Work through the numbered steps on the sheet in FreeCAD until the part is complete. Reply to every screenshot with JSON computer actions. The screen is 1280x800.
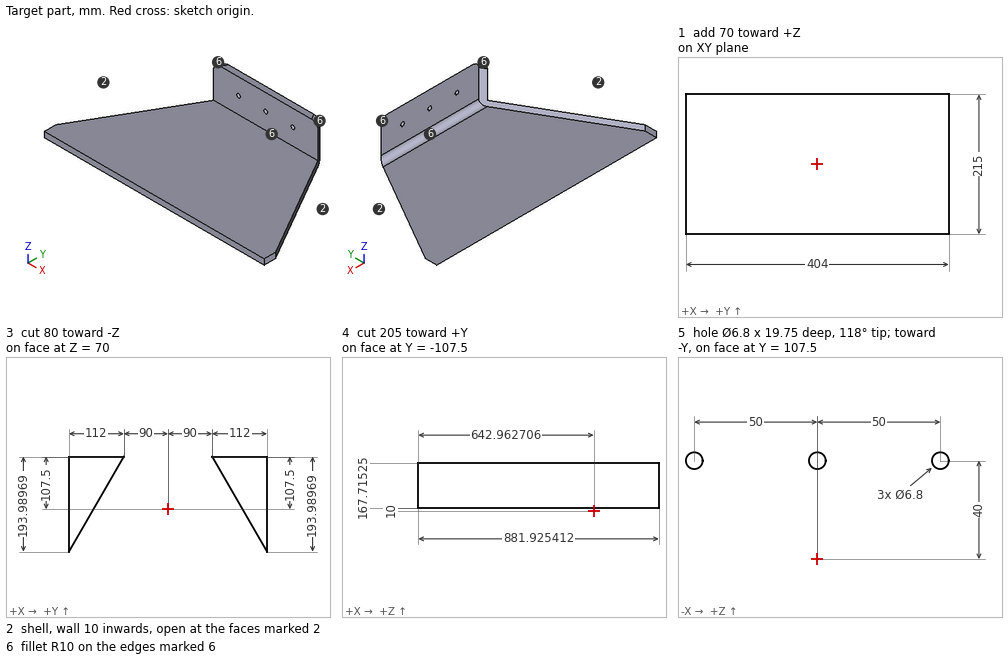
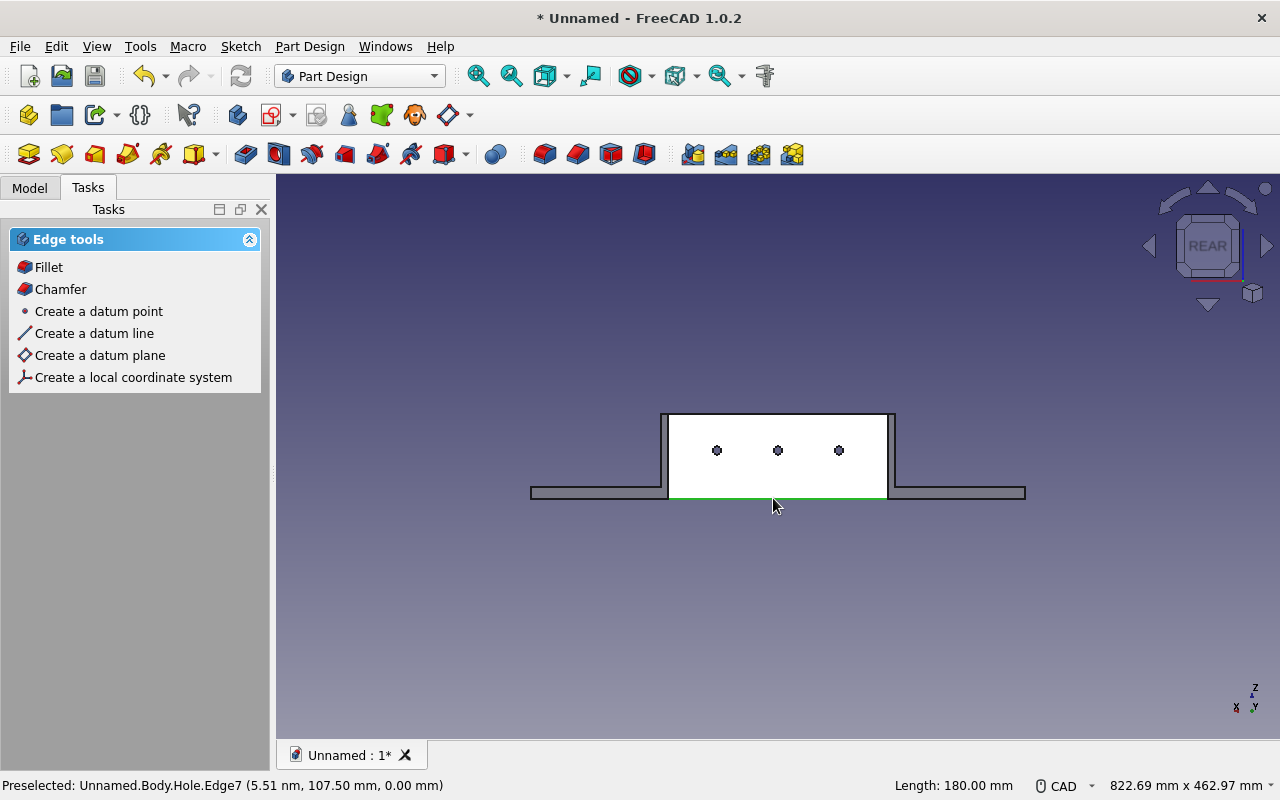
{"action": "scroll", "coordinate": [665, 413], "scroll_direction": "up", "scroll_amount": 6}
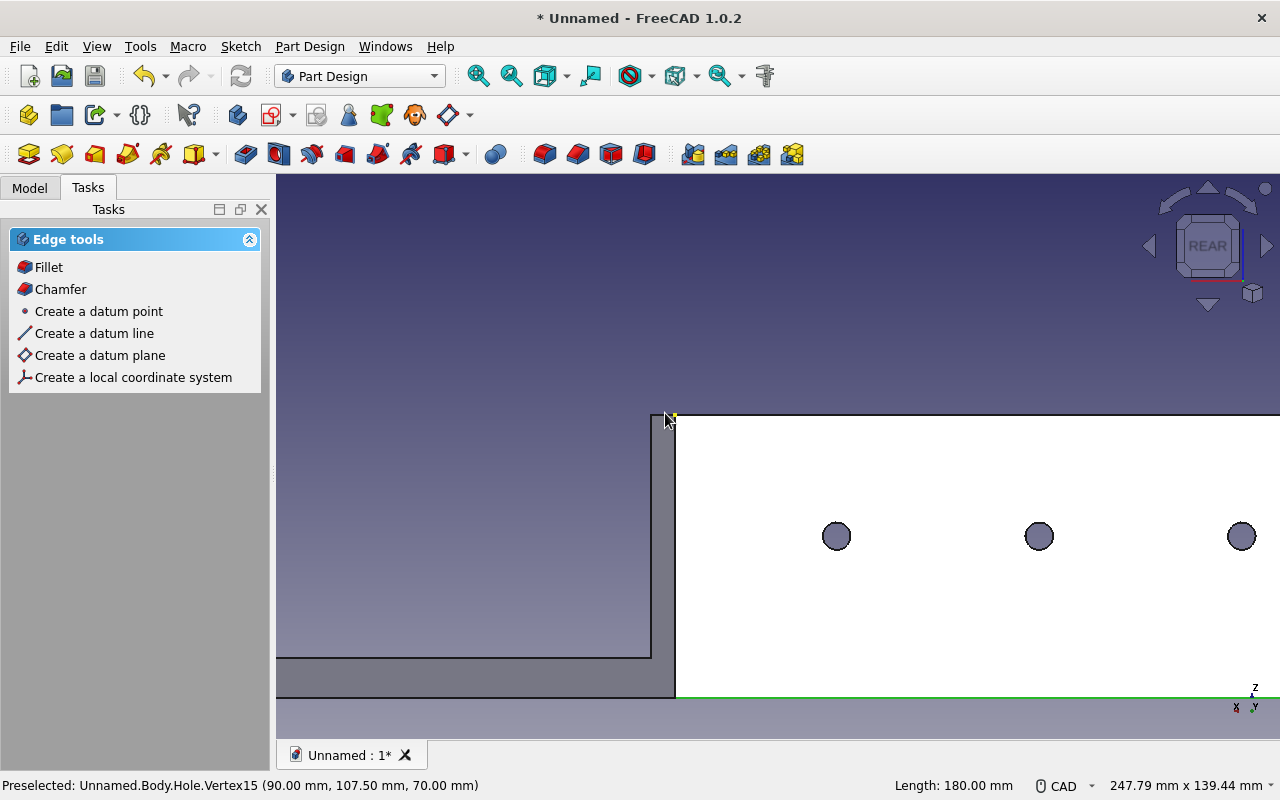
{"action": "left_click", "coordinate": [663, 414], "text": "ctrl"}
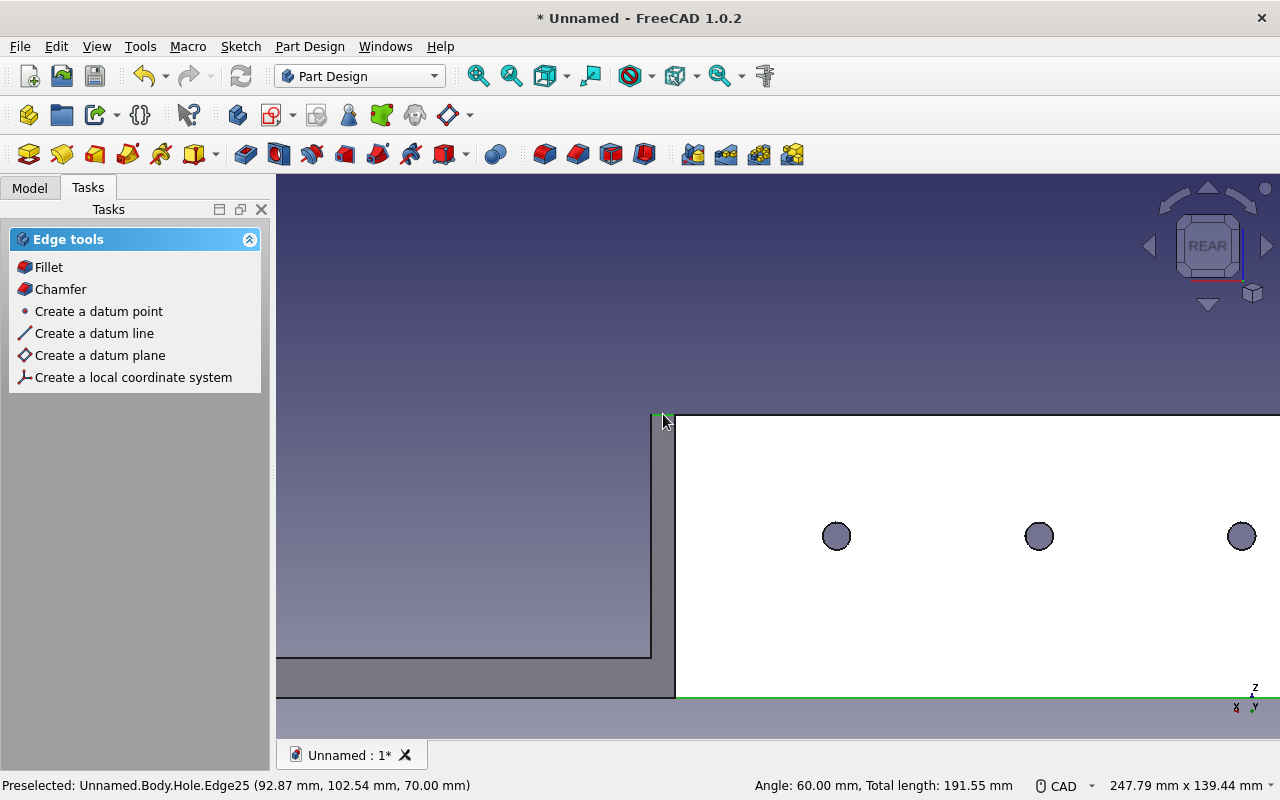
{"action": "left_click", "coordinate": [479, 76]}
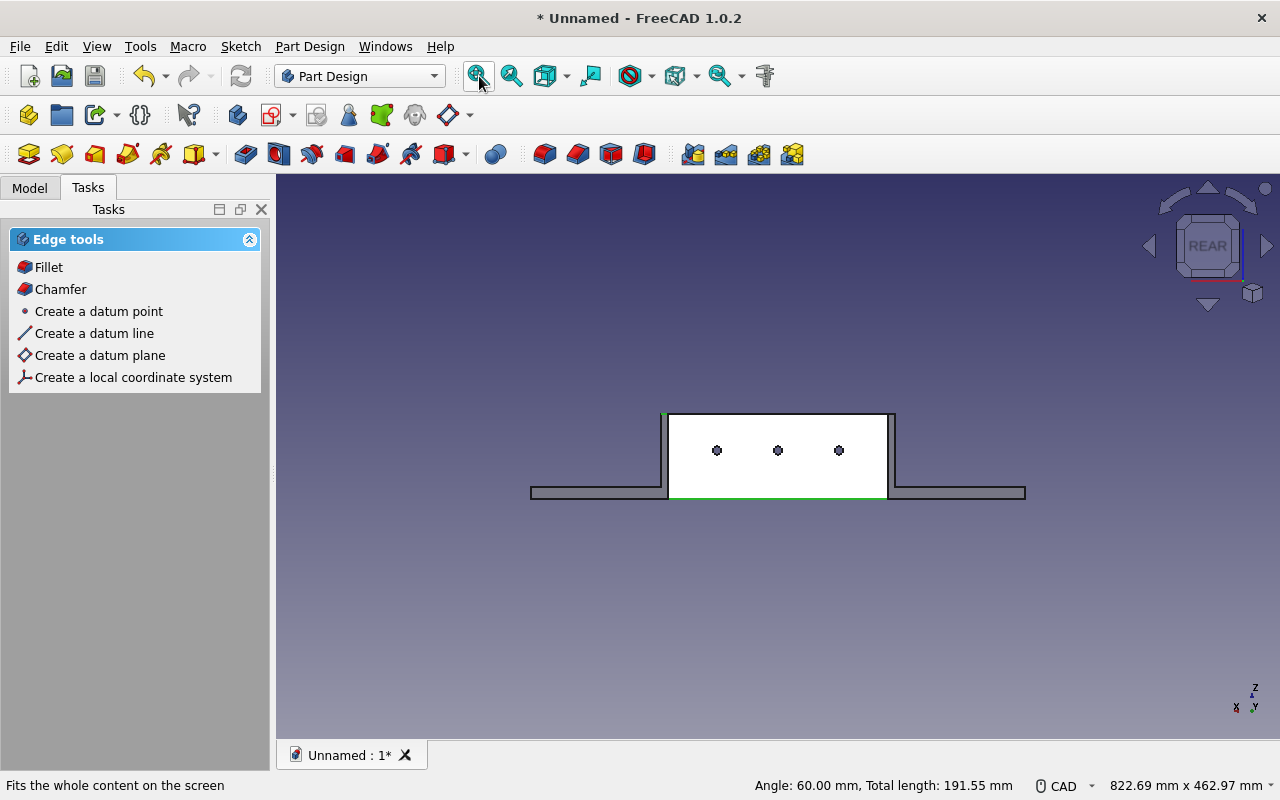
{"action": "key", "text": "0"}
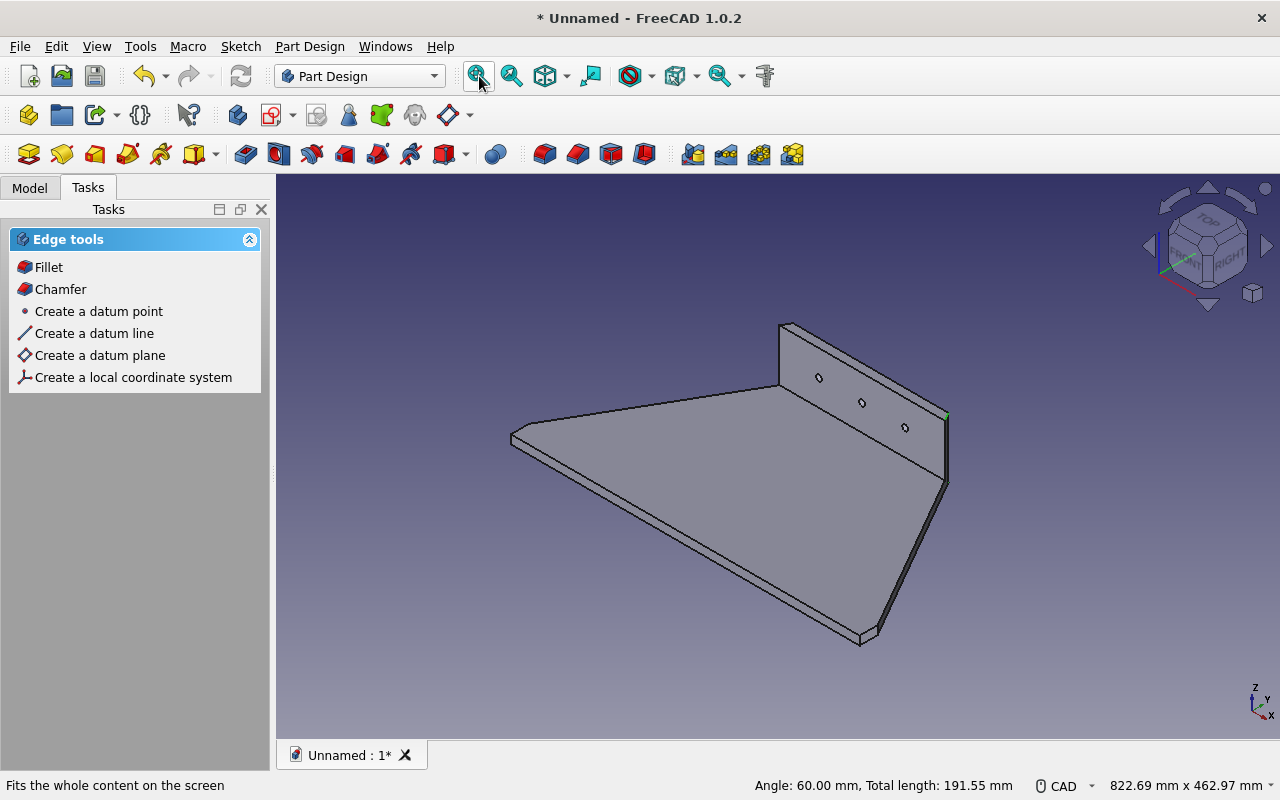
{"action": "scroll", "coordinate": [786, 323], "scroll_direction": "up", "scroll_amount": 6}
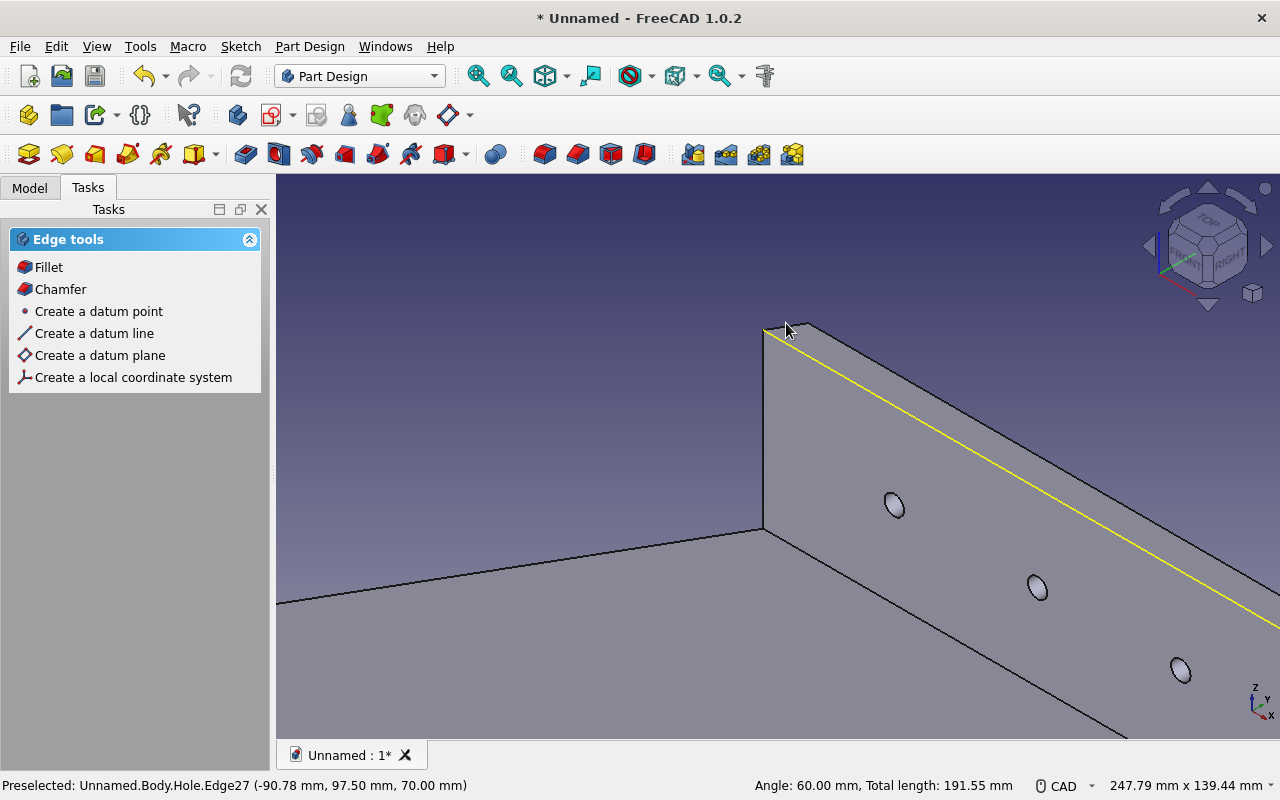
{"action": "left_click", "coordinate": [479, 76]}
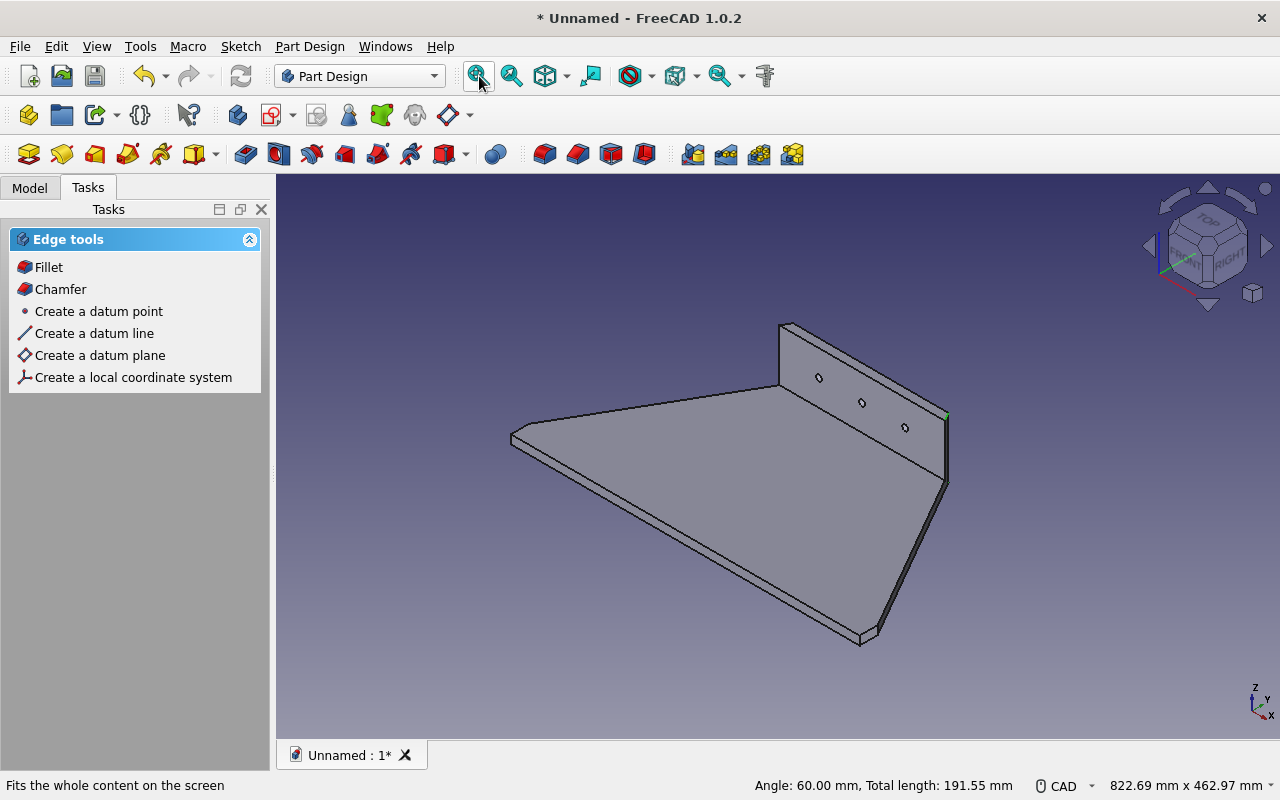
{"action": "key", "text": "2"}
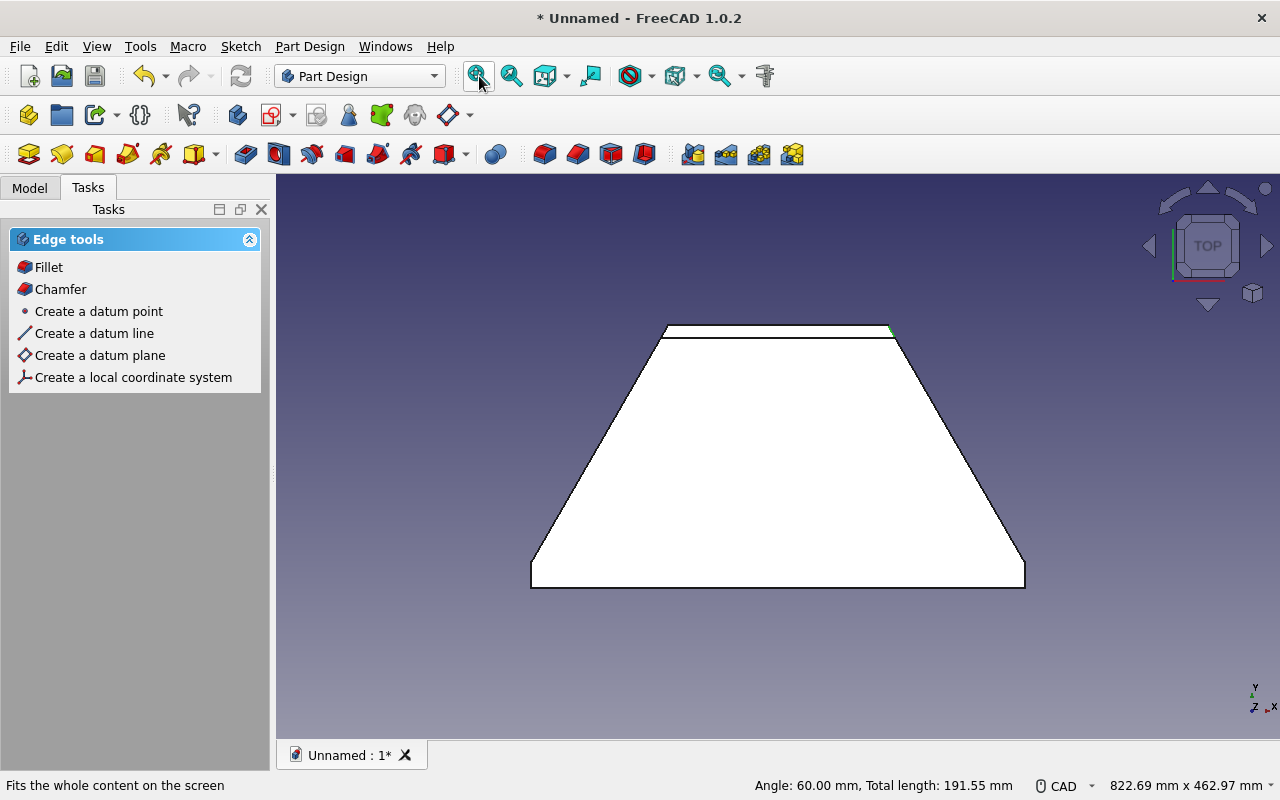
{"action": "left_click", "coordinate": [665, 330], "text": "ctrl"}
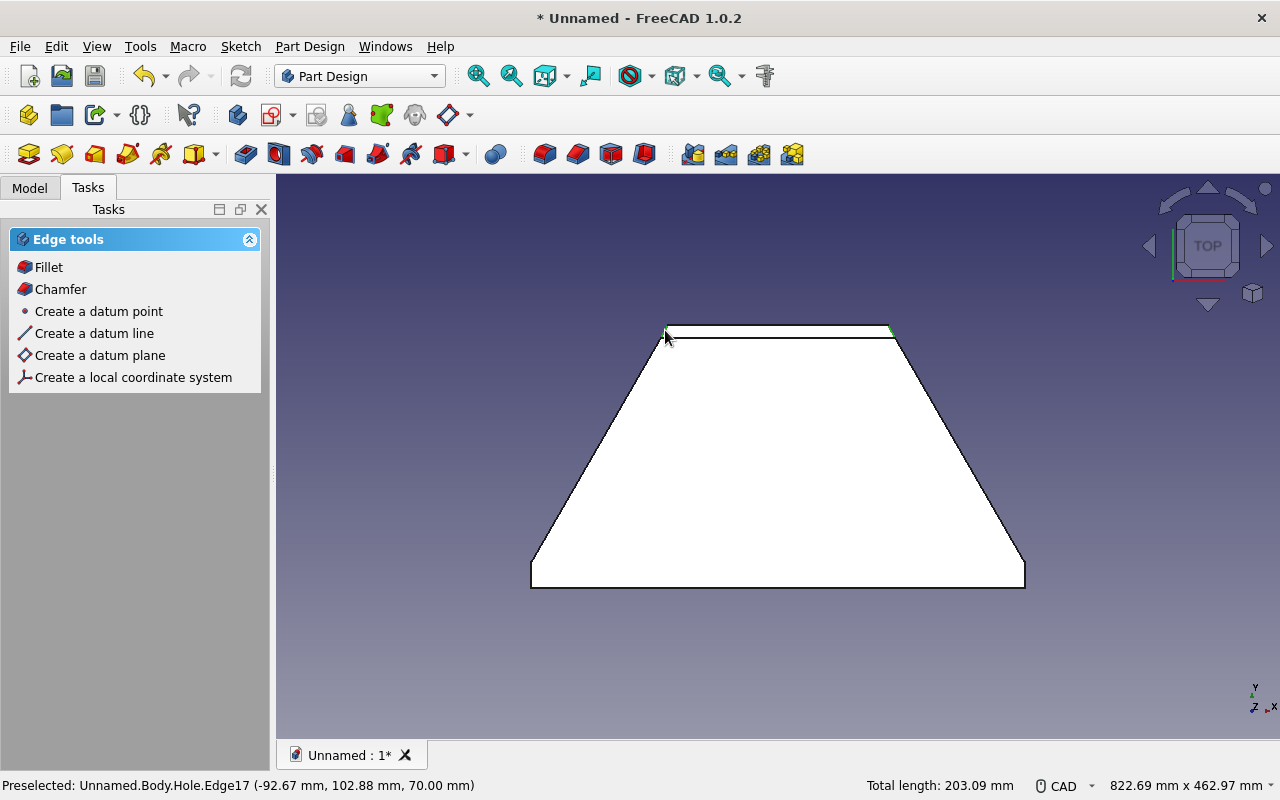
{"action": "left_click", "coordinate": [545, 154]}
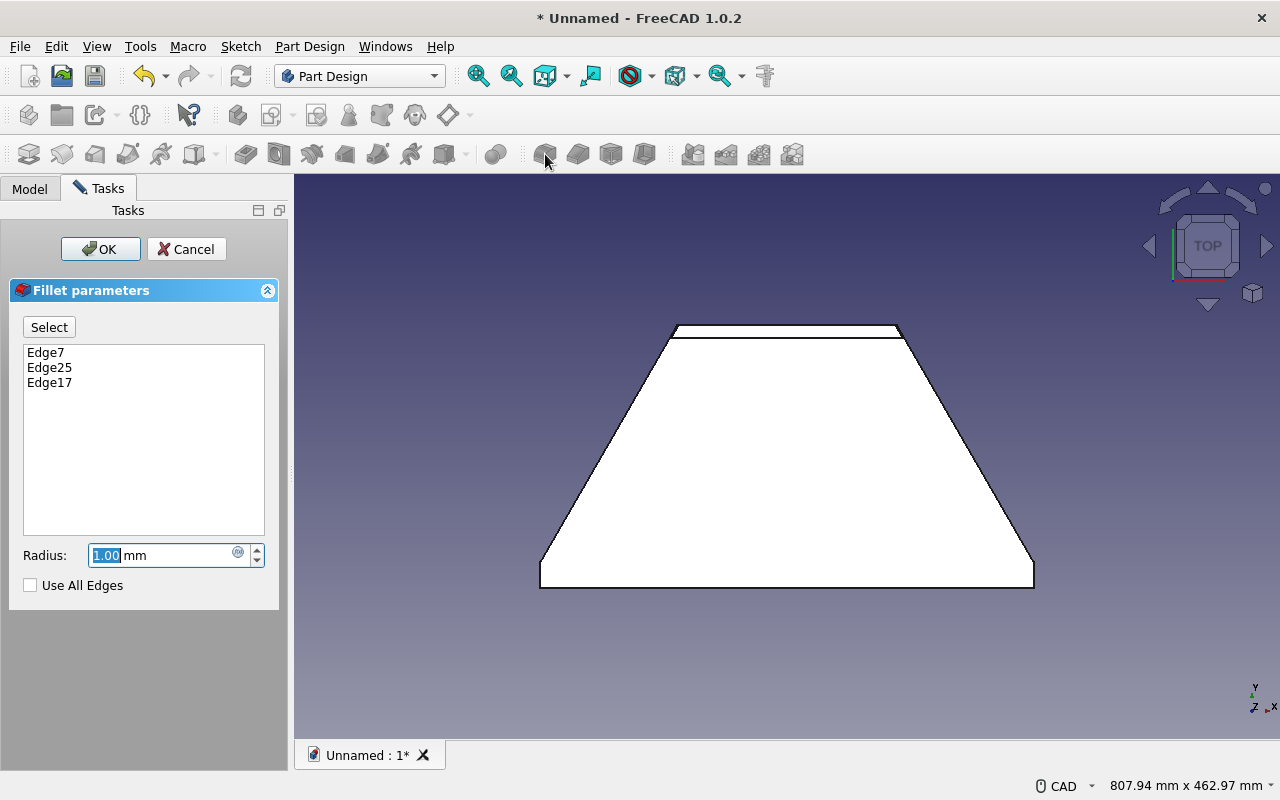
{"action": "type", "text": "10"}
{"action": "key", "text": "Tab"}